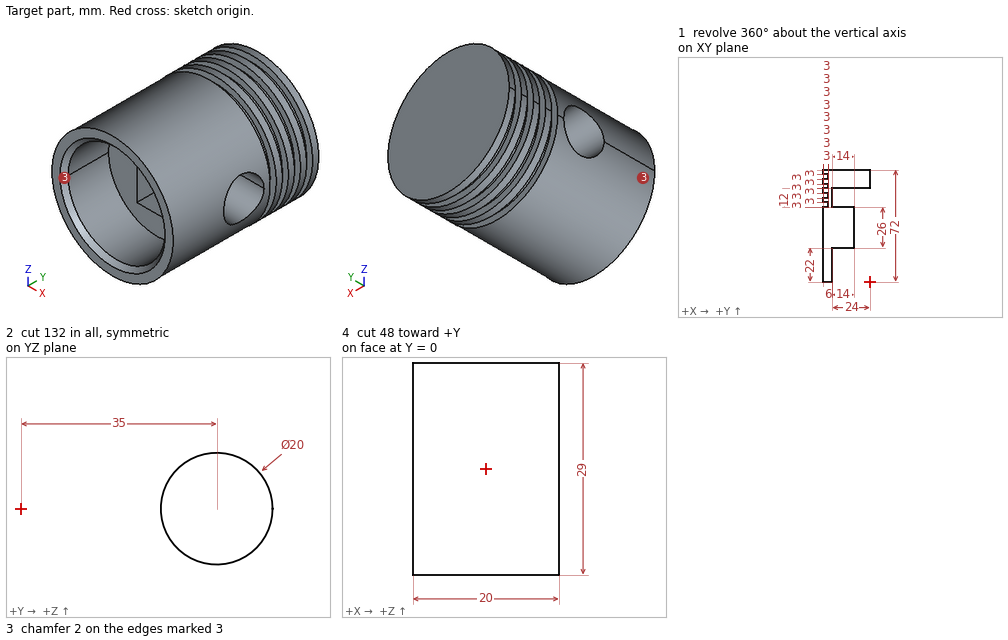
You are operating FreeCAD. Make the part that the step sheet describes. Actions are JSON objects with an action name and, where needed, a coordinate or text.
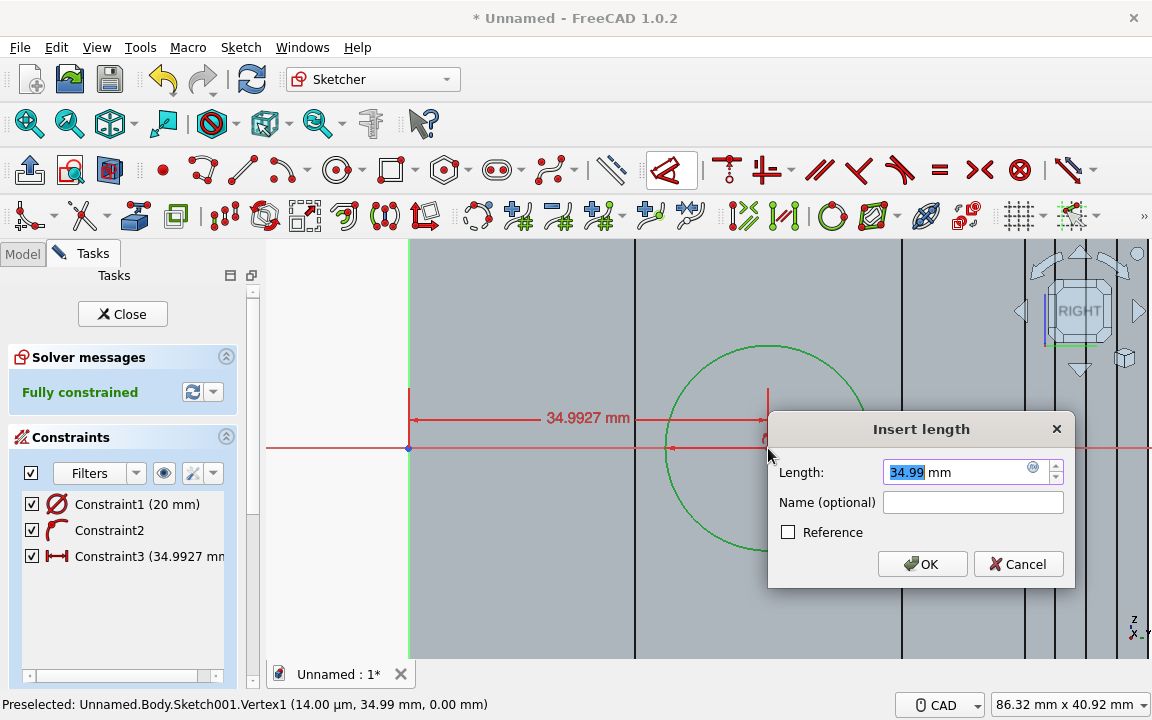
{"action": "type", "text": "35"}
{"action": "key", "text": "Return"}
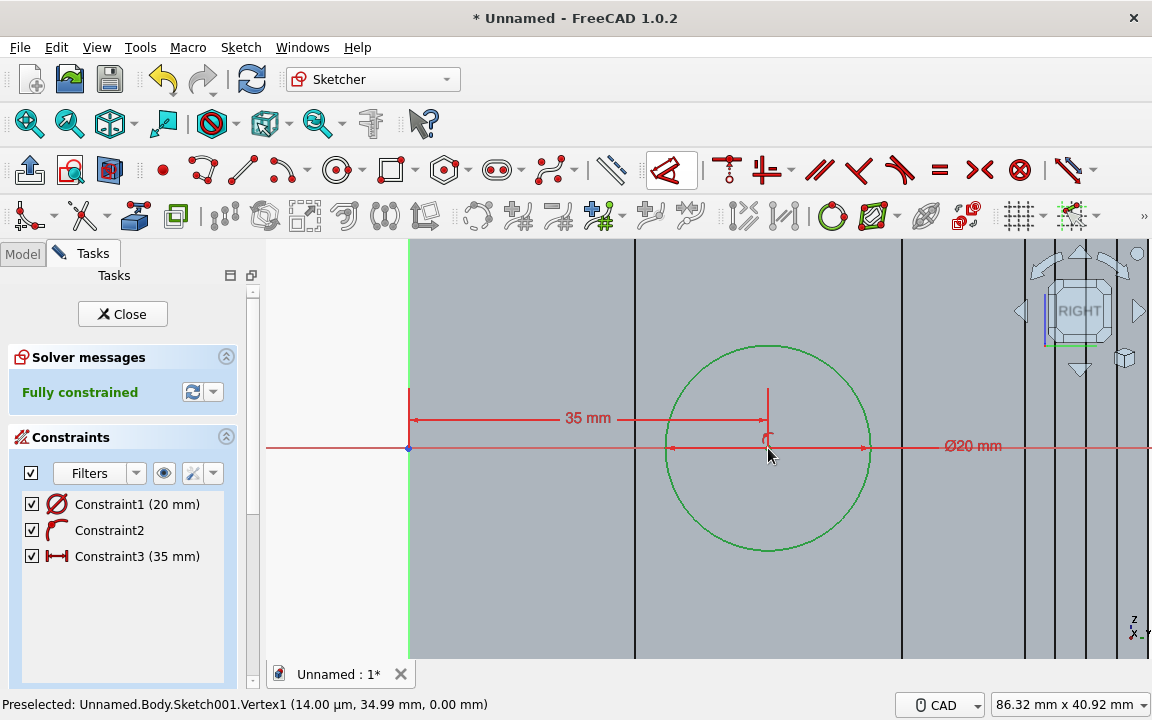
{"action": "left_click", "coordinate": [123, 314]}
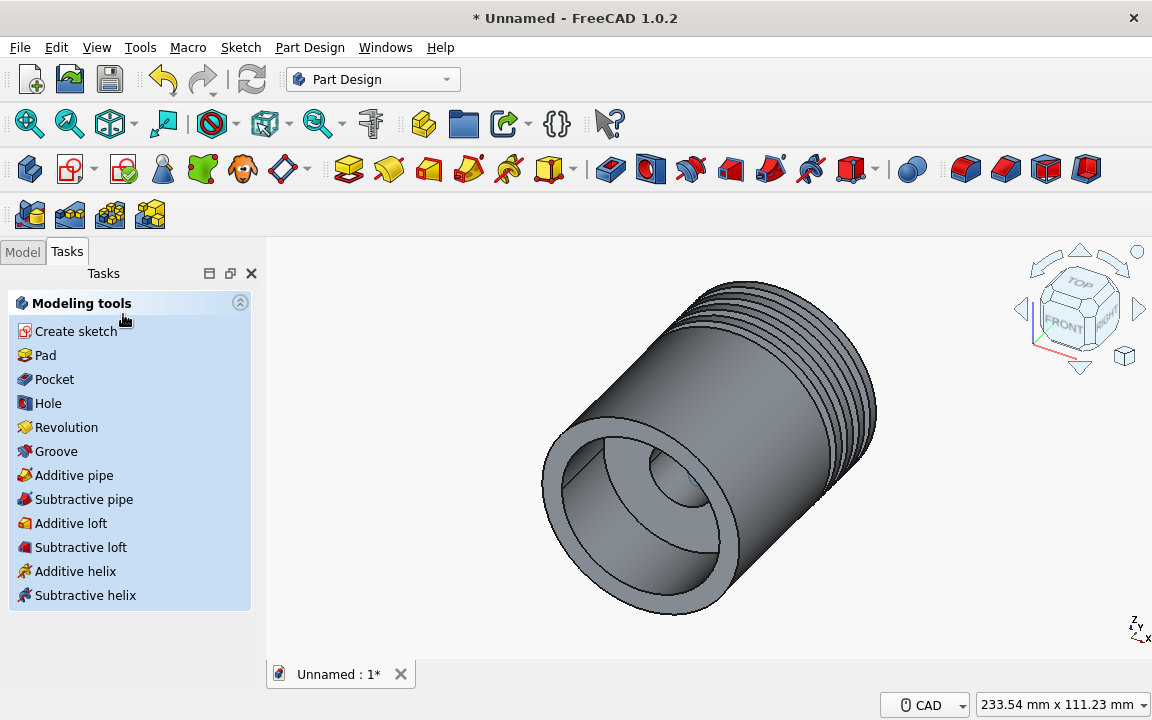
{"action": "left_click", "coordinate": [612, 170]}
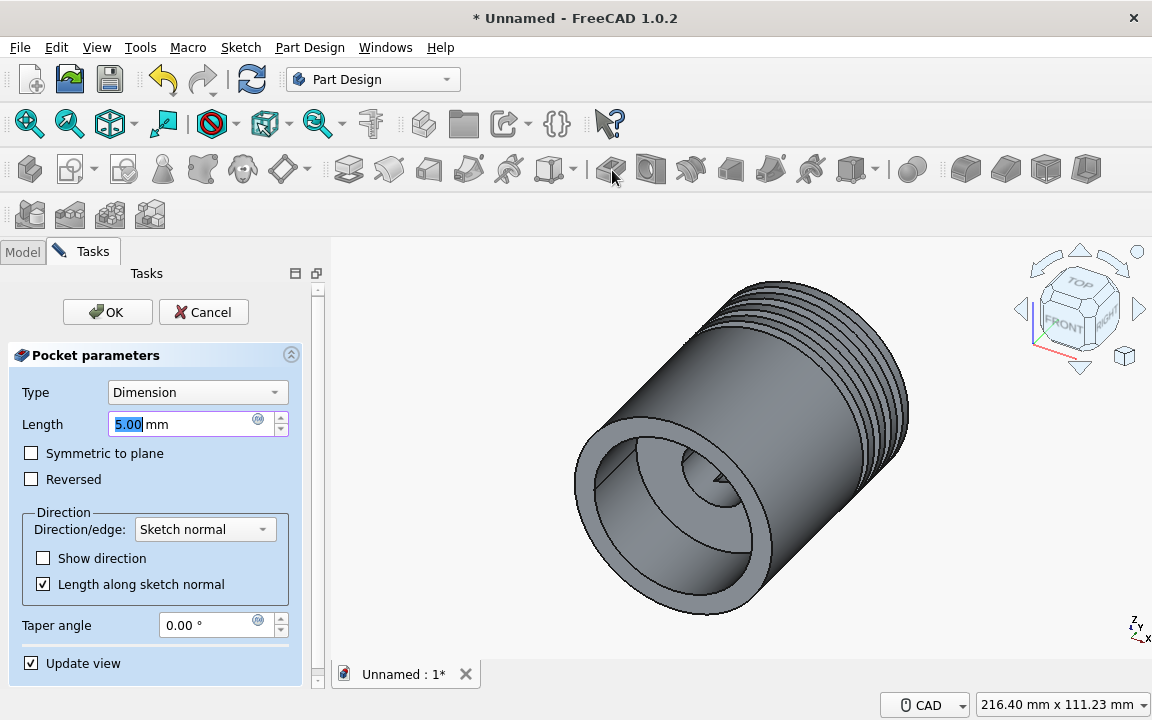
{"action": "type", "text": "132"}
{"action": "key", "text": "Tab"}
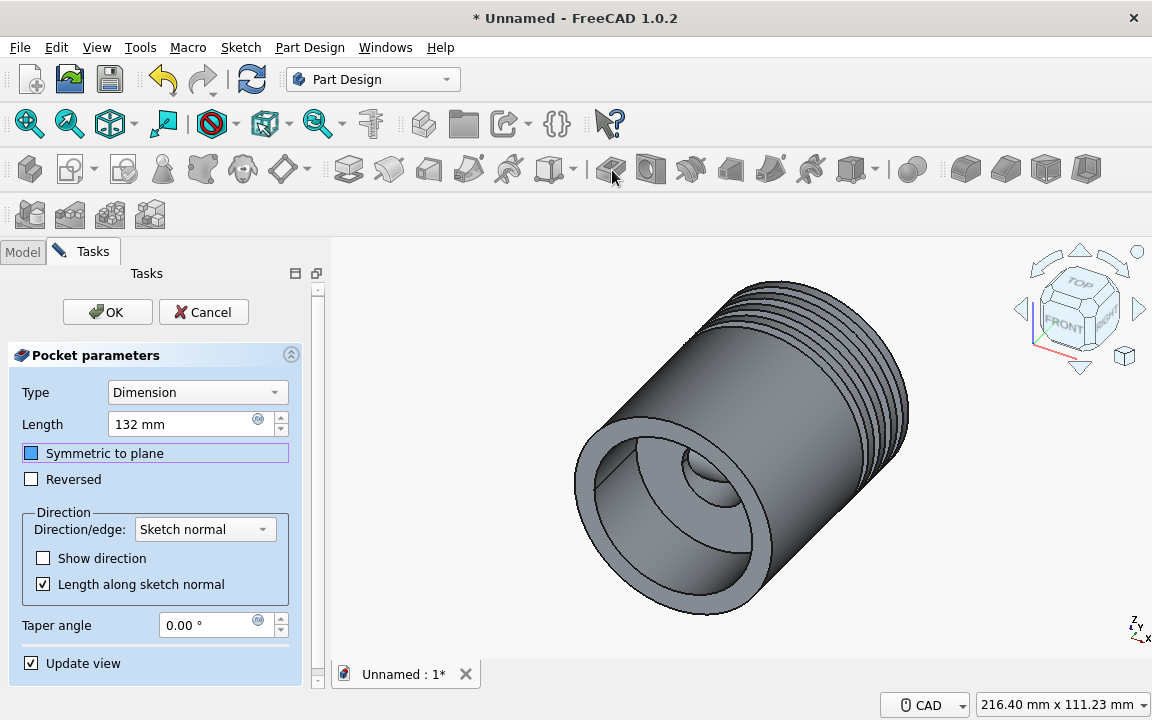
{"action": "left_click", "coordinate": [30, 453]}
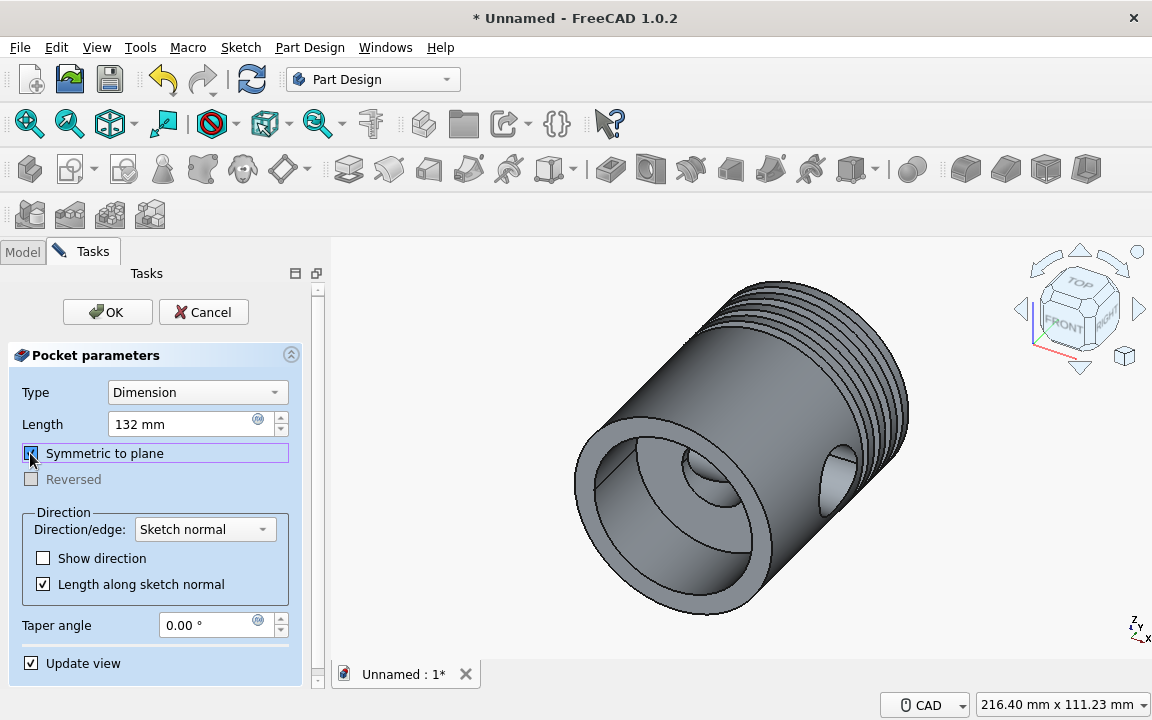
{"action": "left_click", "coordinate": [108, 312]}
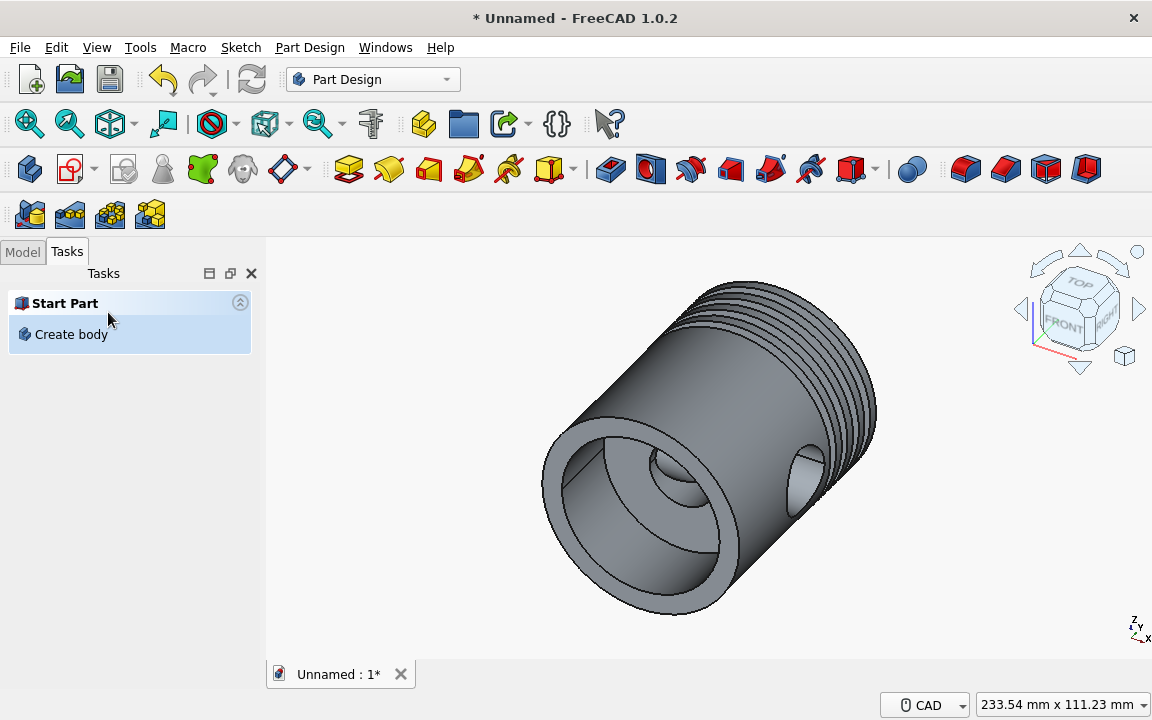
{"action": "left_click", "coordinate": [705, 580]}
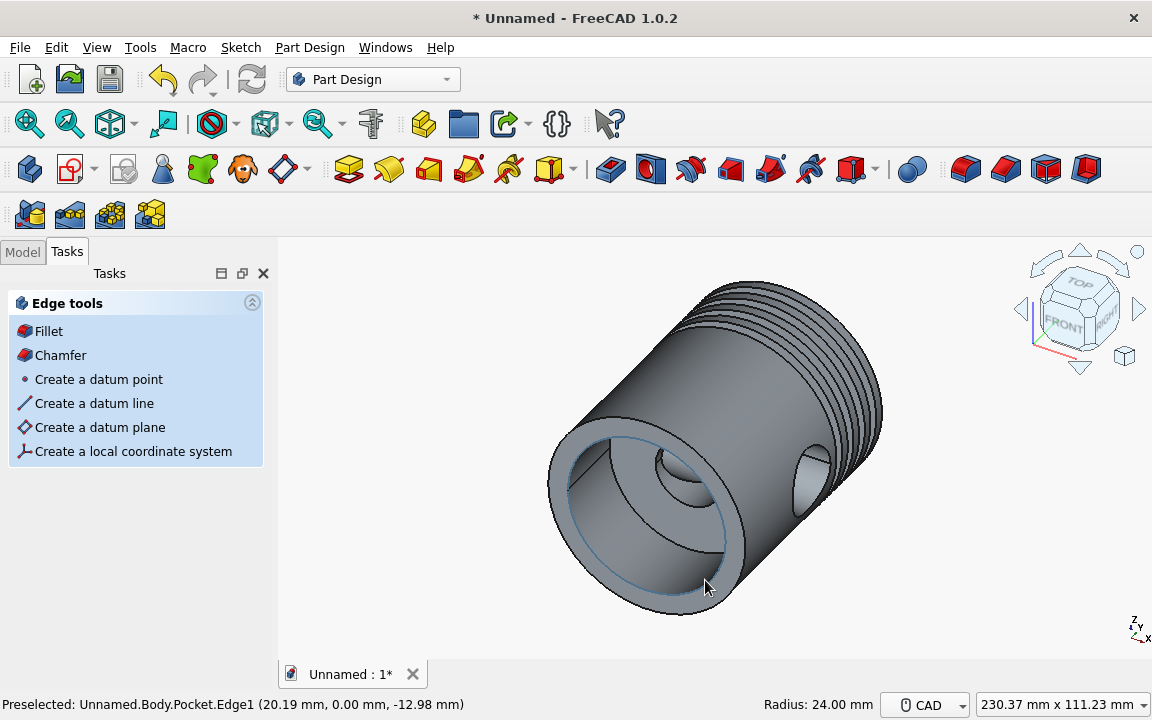
{"action": "left_click", "coordinate": [1006, 170]}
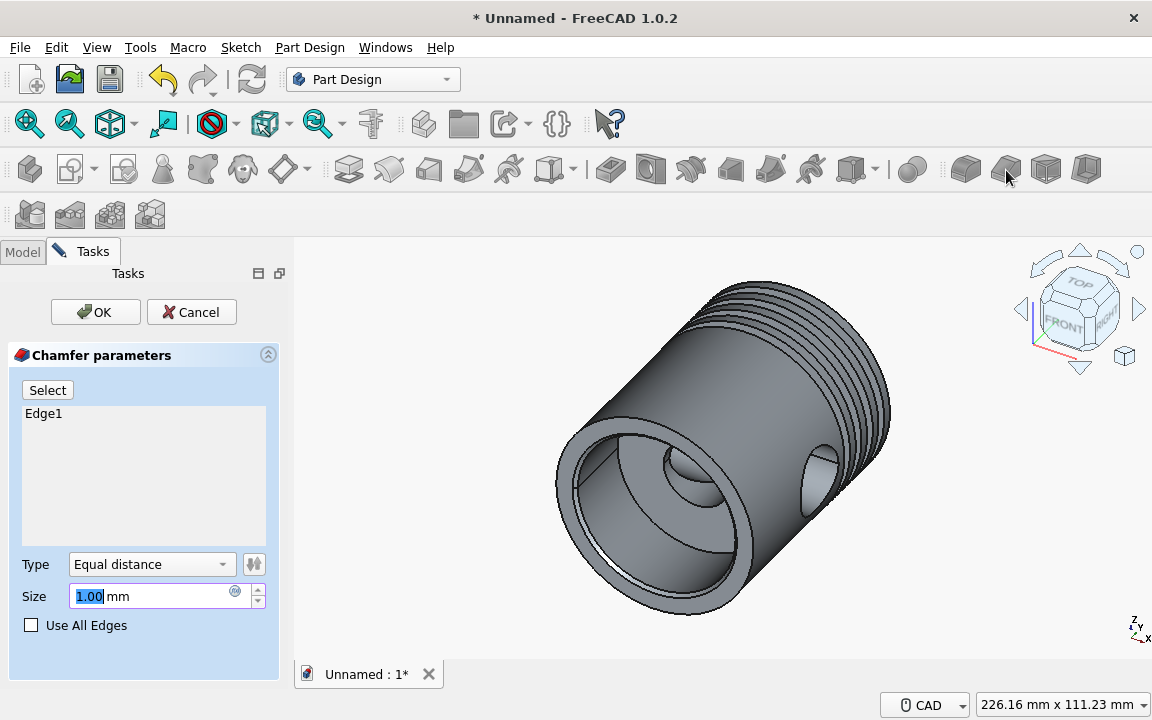
{"action": "type", "text": "2"}
{"action": "key", "text": "Tab"}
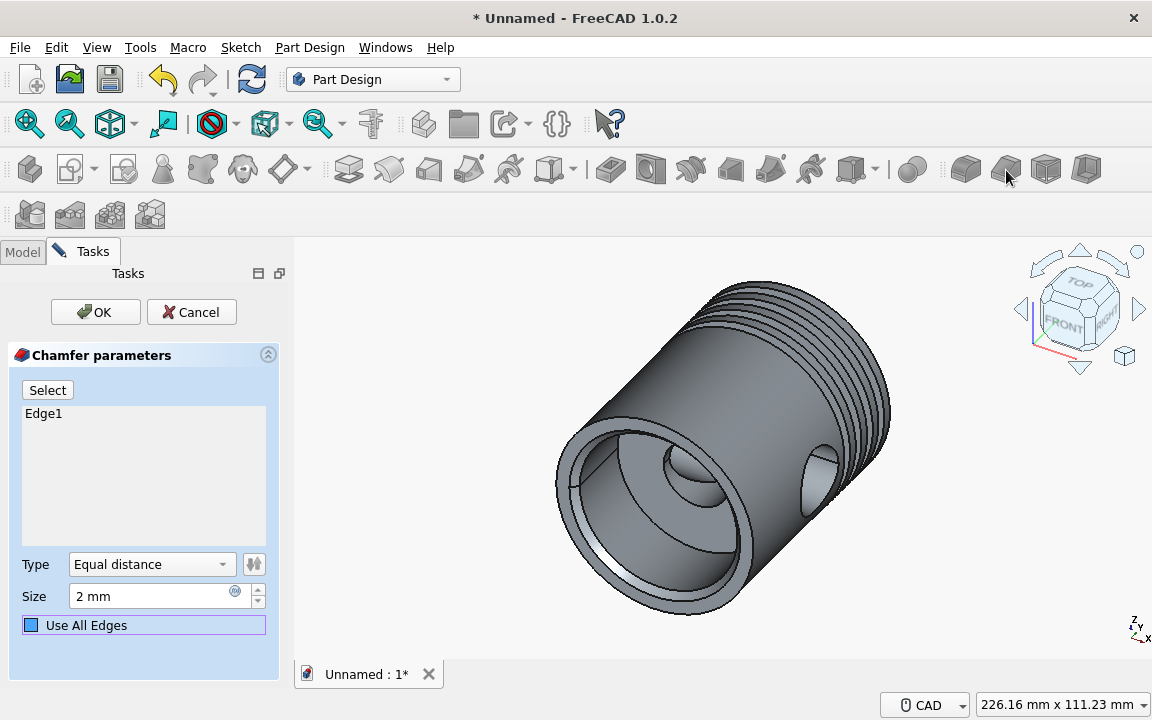
{"action": "left_click", "coordinate": [96, 312]}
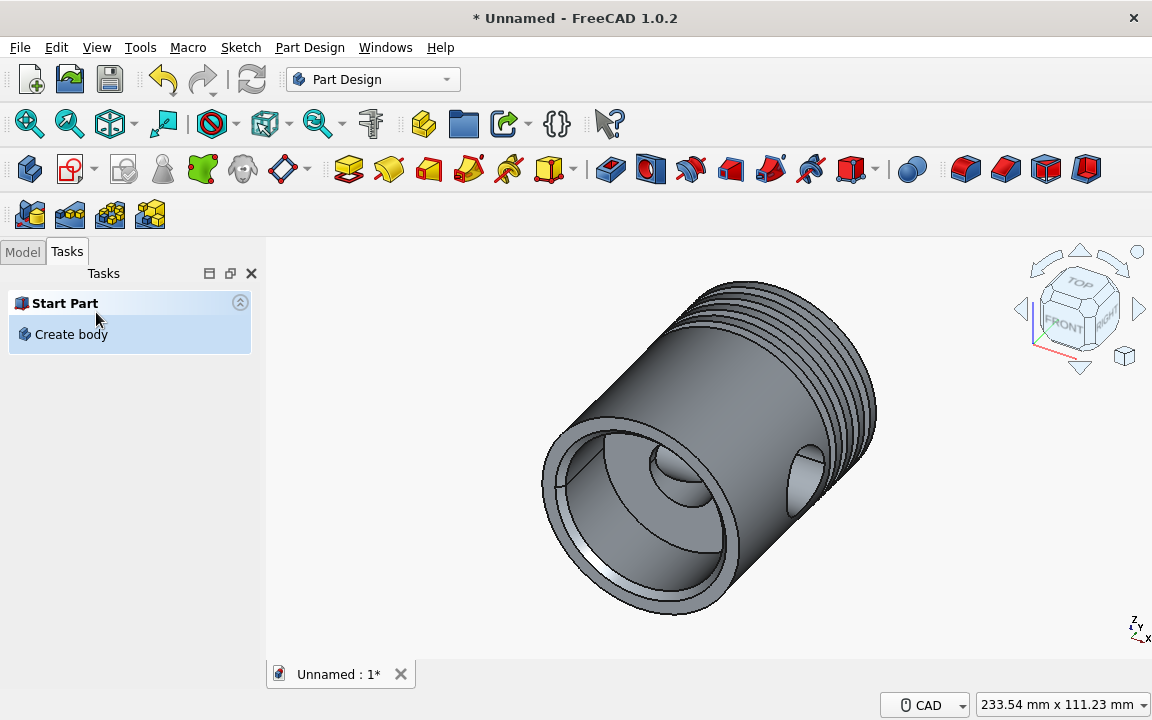
{"action": "left_click", "coordinate": [613, 426]}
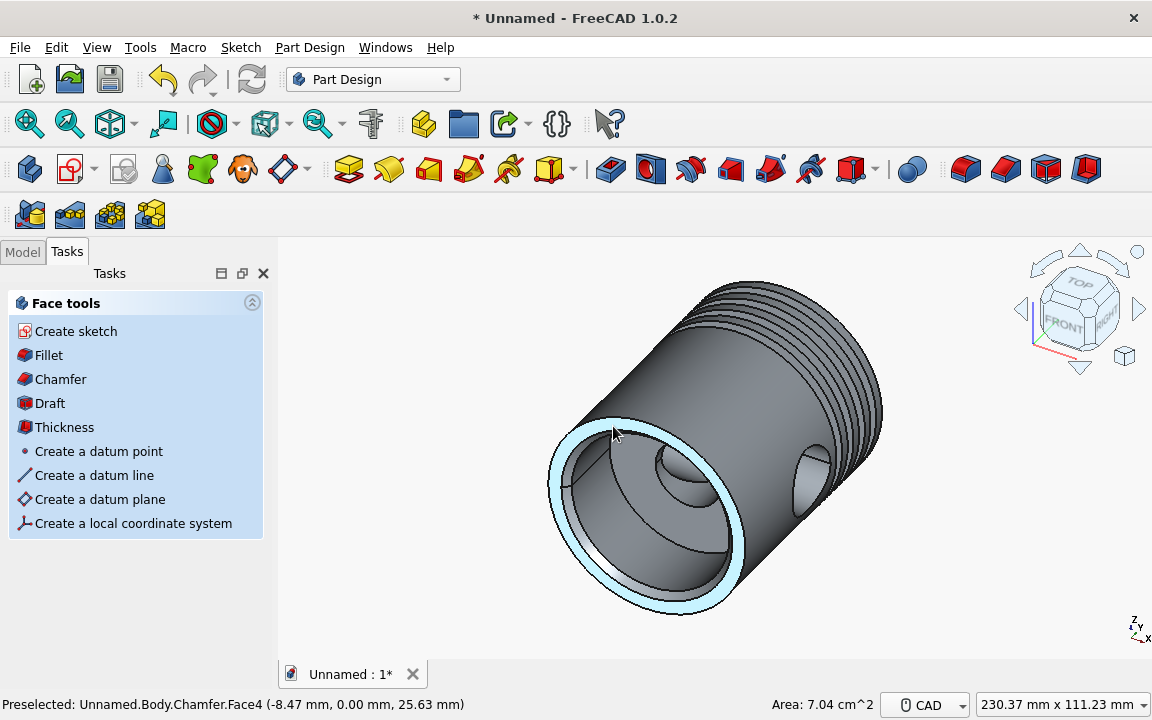
{"action": "left_click", "coordinate": [70, 170]}